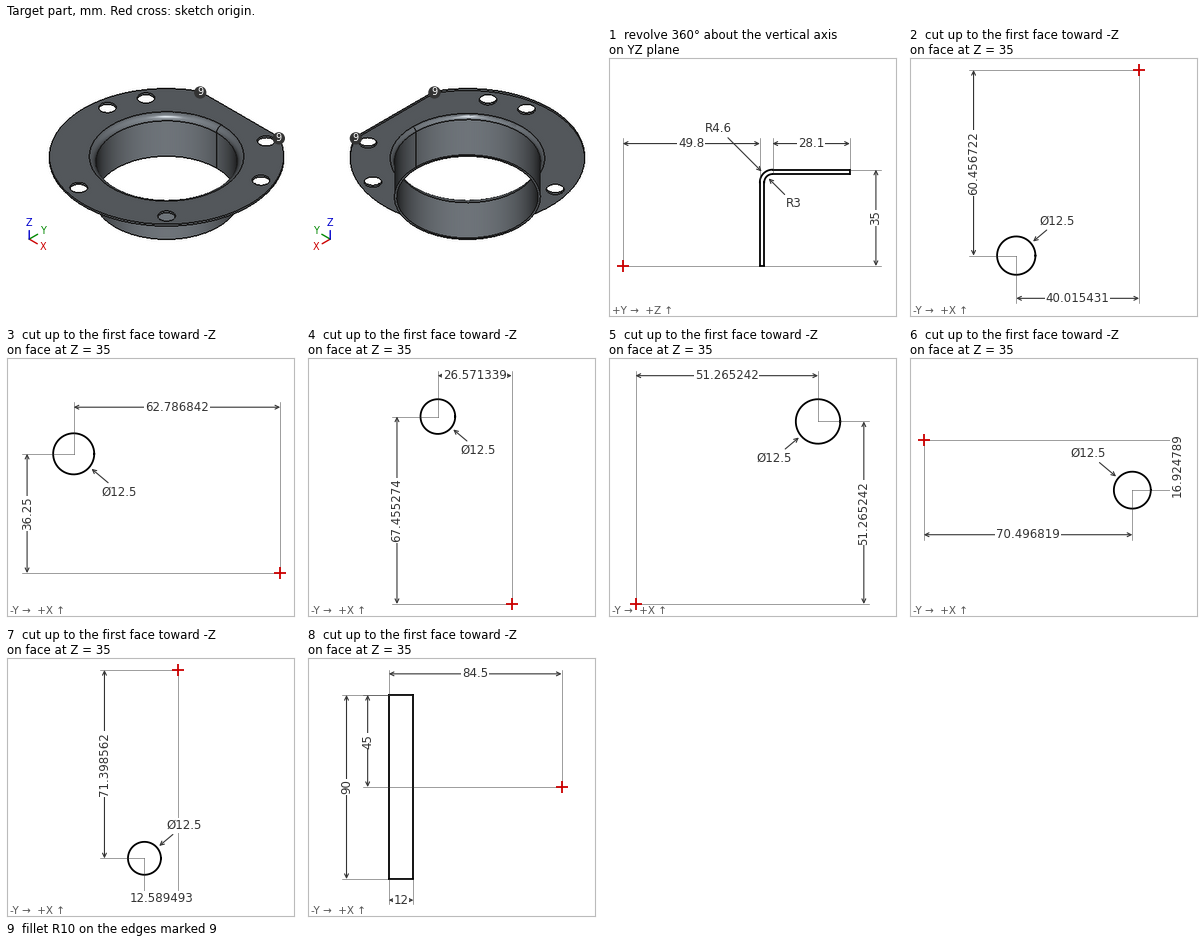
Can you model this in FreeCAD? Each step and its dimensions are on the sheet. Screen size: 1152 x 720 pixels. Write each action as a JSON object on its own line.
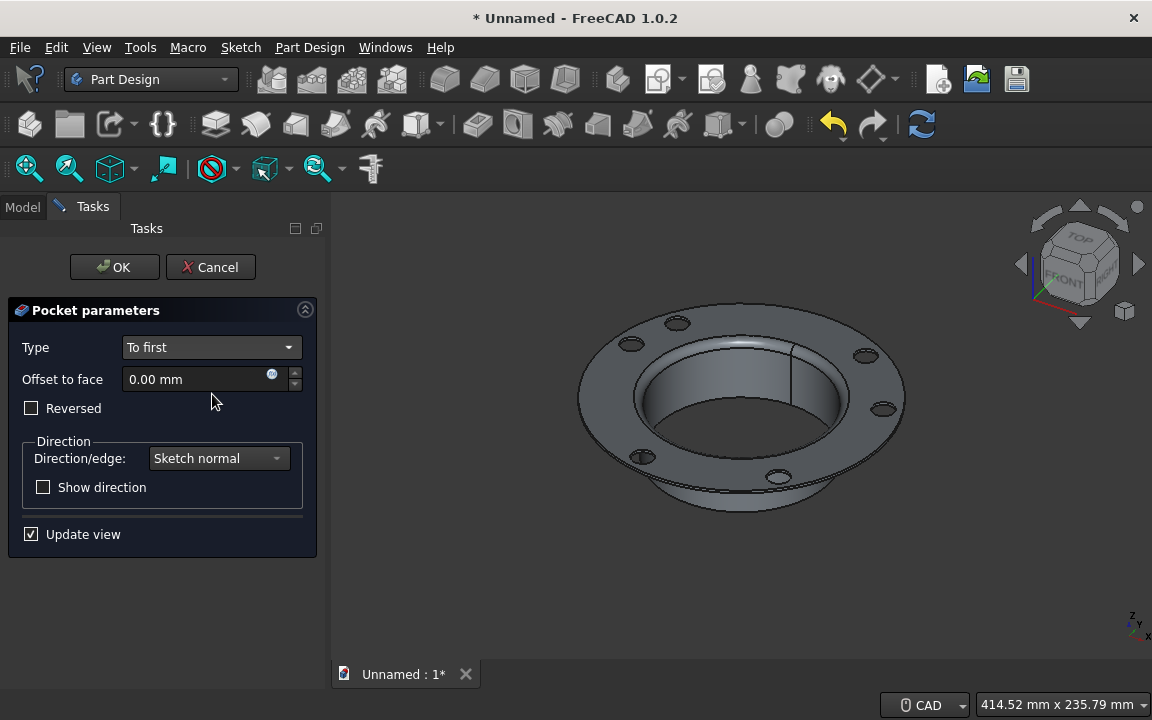
{"action": "left_click", "coordinate": [115, 267]}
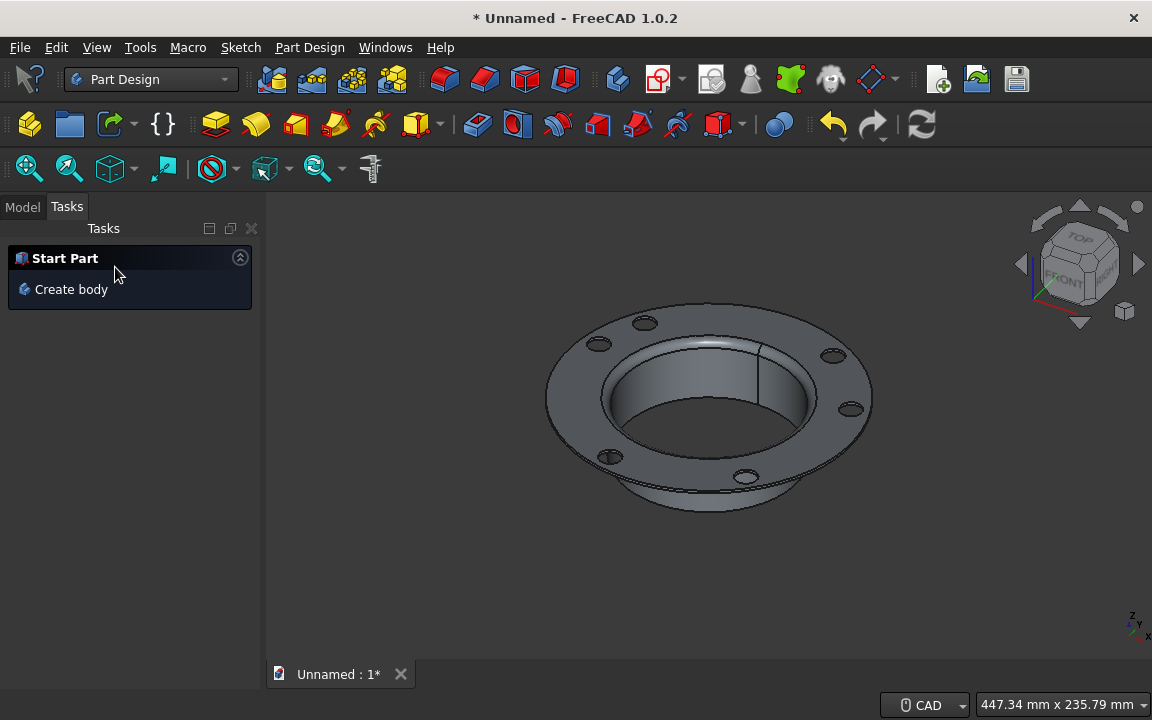
{"action": "left_click", "coordinate": [837, 377]}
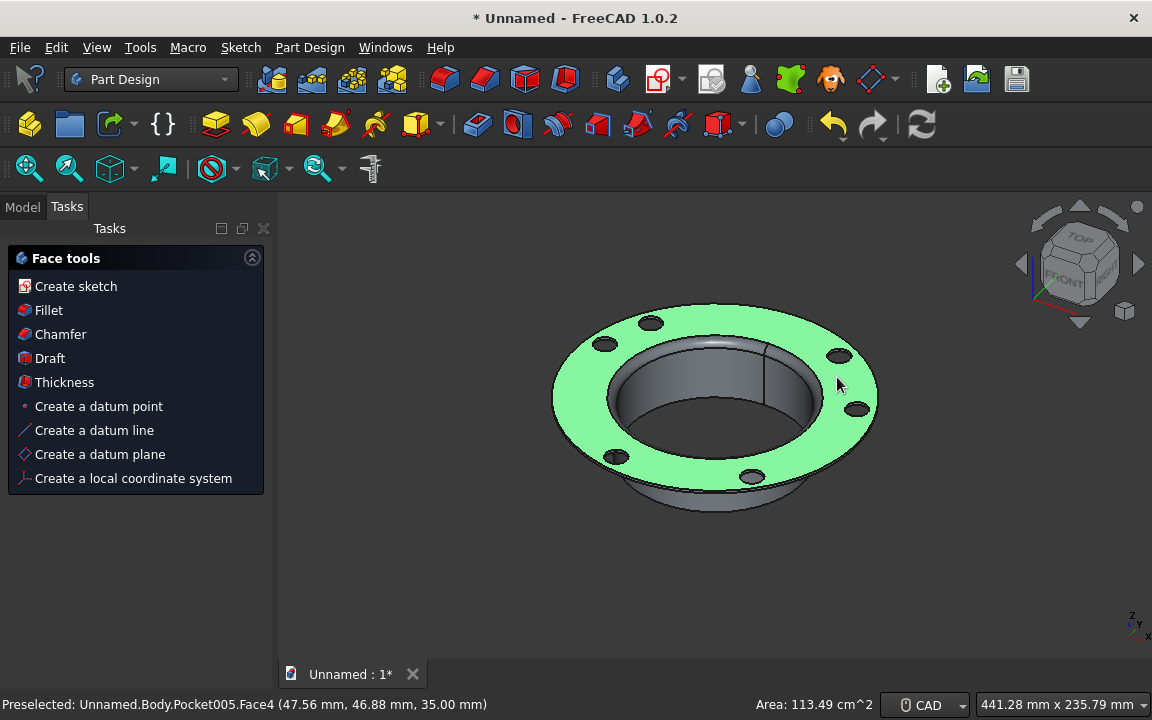
{"action": "left_click", "coordinate": [658, 80]}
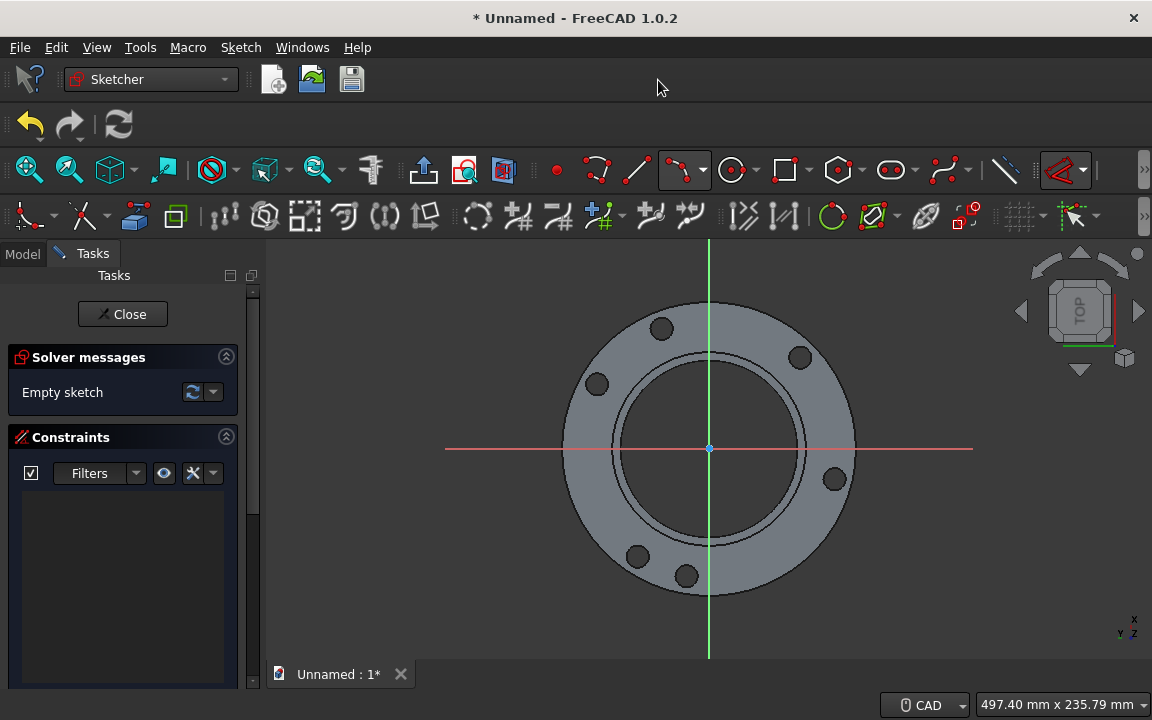
{"action": "scroll", "coordinate": [620, 449], "scroll_direction": "up", "scroll_amount": 2}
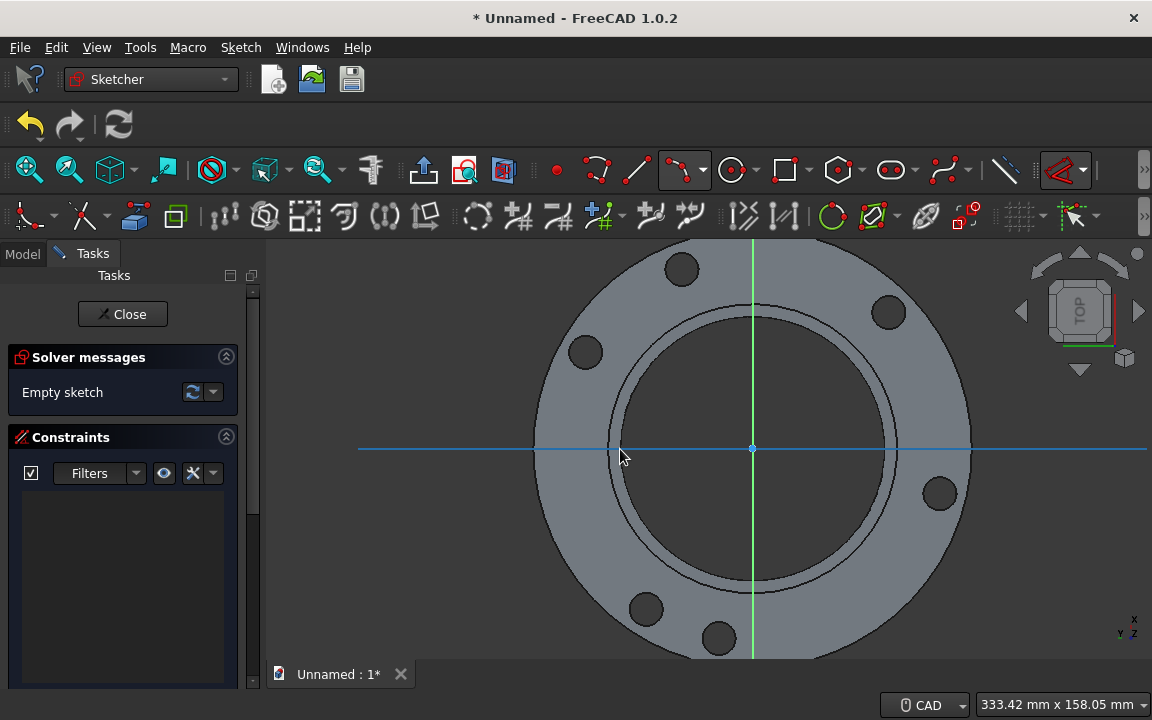
{"action": "key", "text": "g r"}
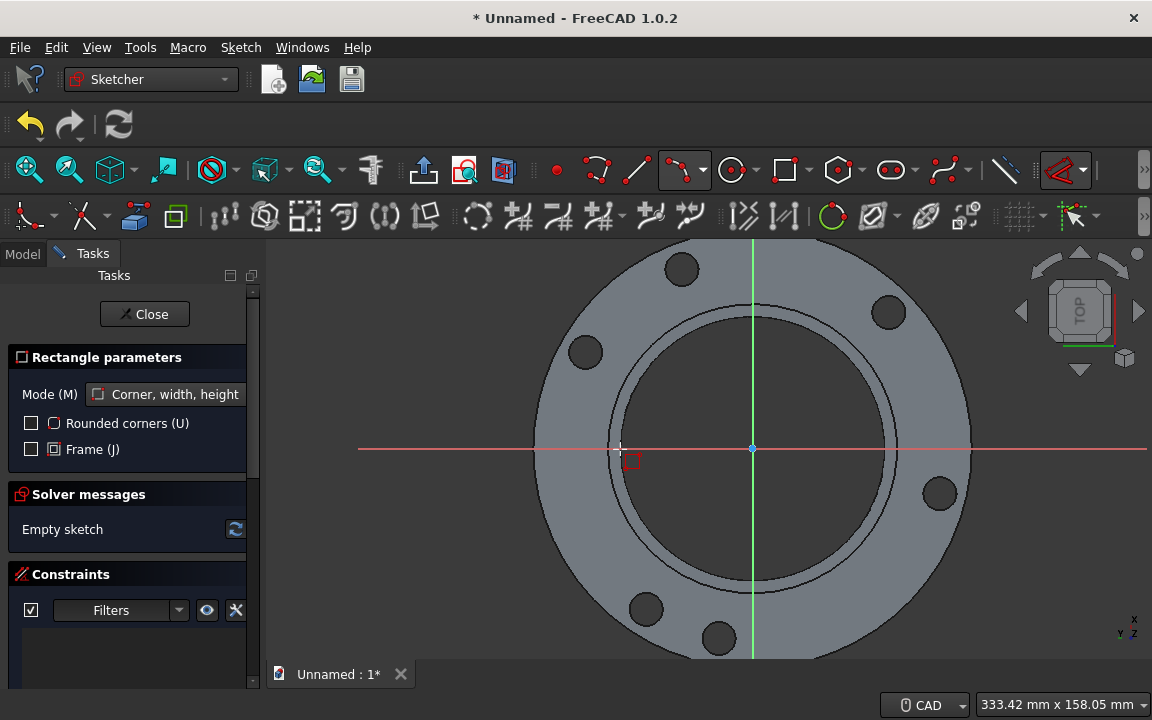
{"action": "left_click", "coordinate": [528, 329]}
{"action": "mouse_move", "coordinate": [560, 568]}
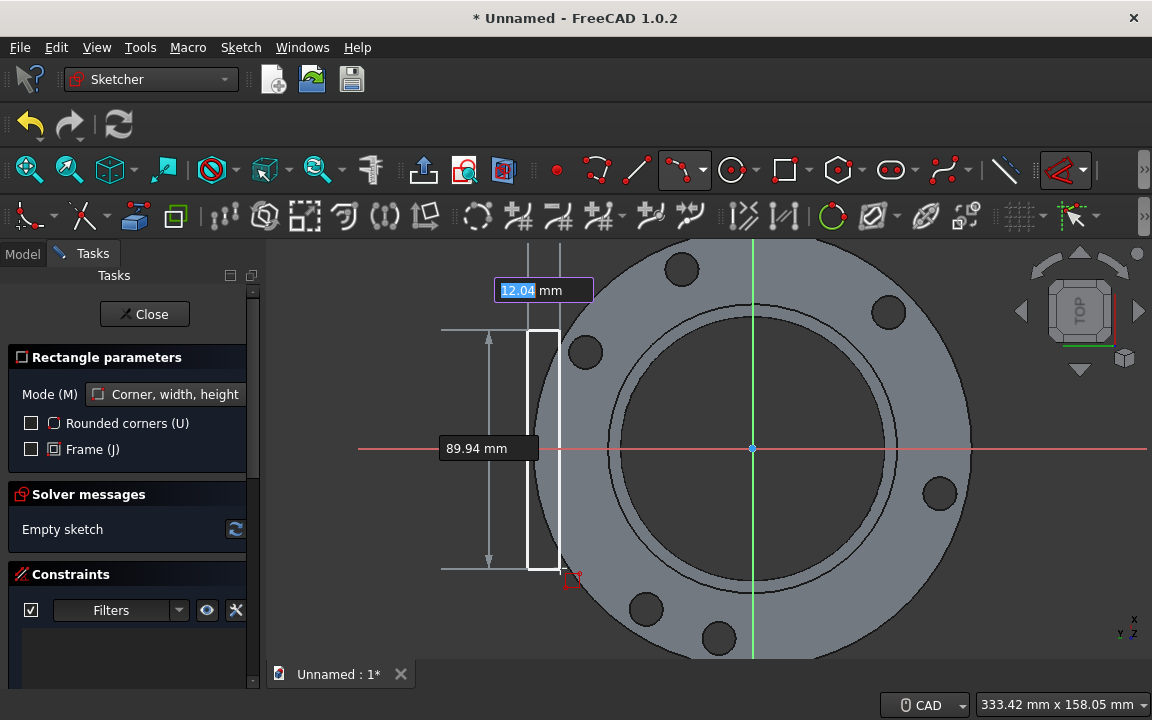
{"action": "type", "text": "12"}
{"action": "key", "text": "Tab"}
{"action": "type", "text": "90"}
{"action": "key", "text": "Return"}
{"action": "key", "text": "Escape"}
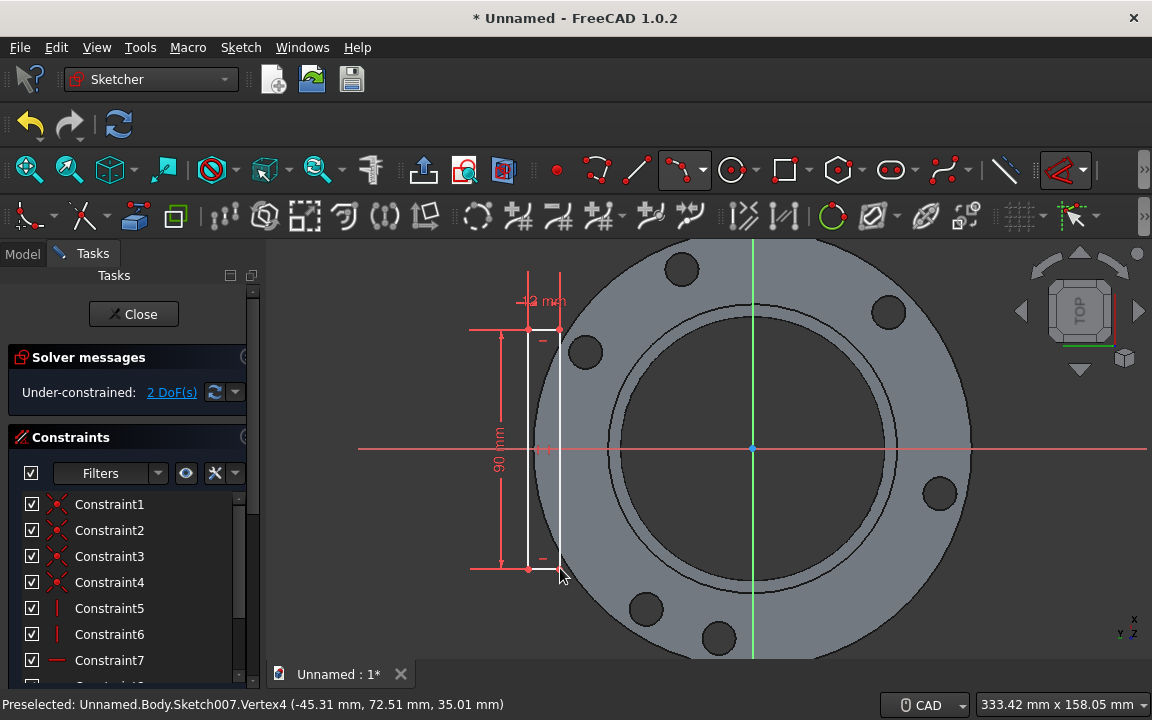
{"action": "left_click", "coordinate": [528, 330]}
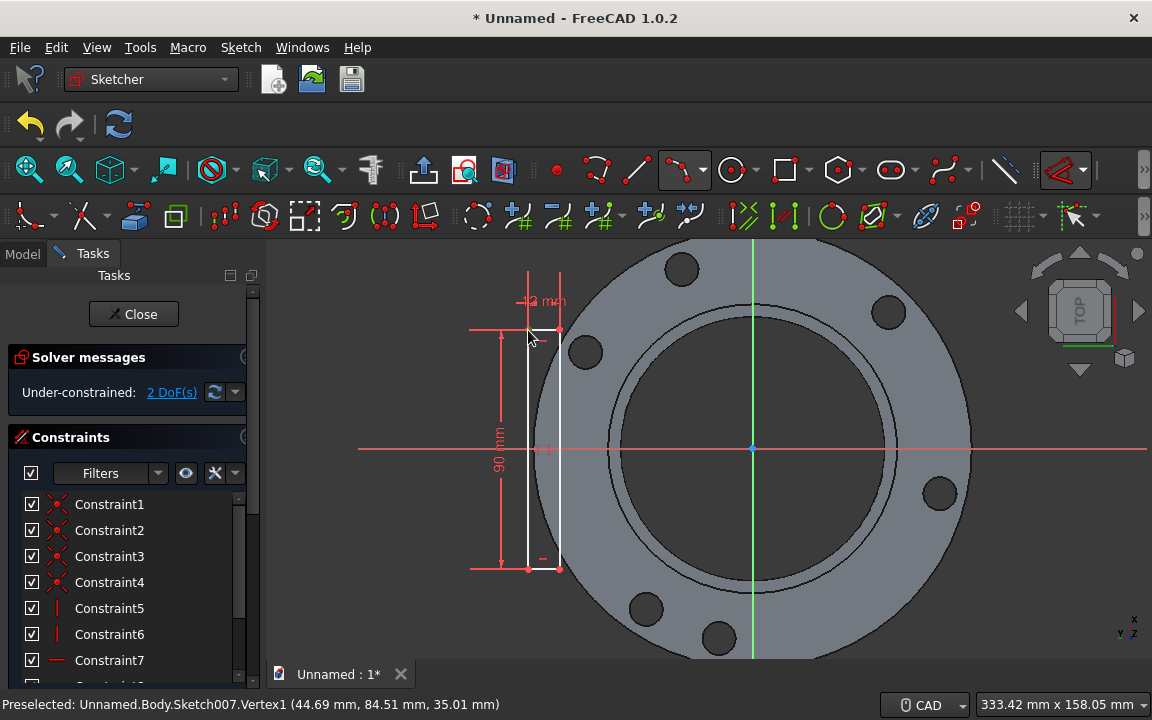
{"action": "left_click", "coordinate": [1086, 170]}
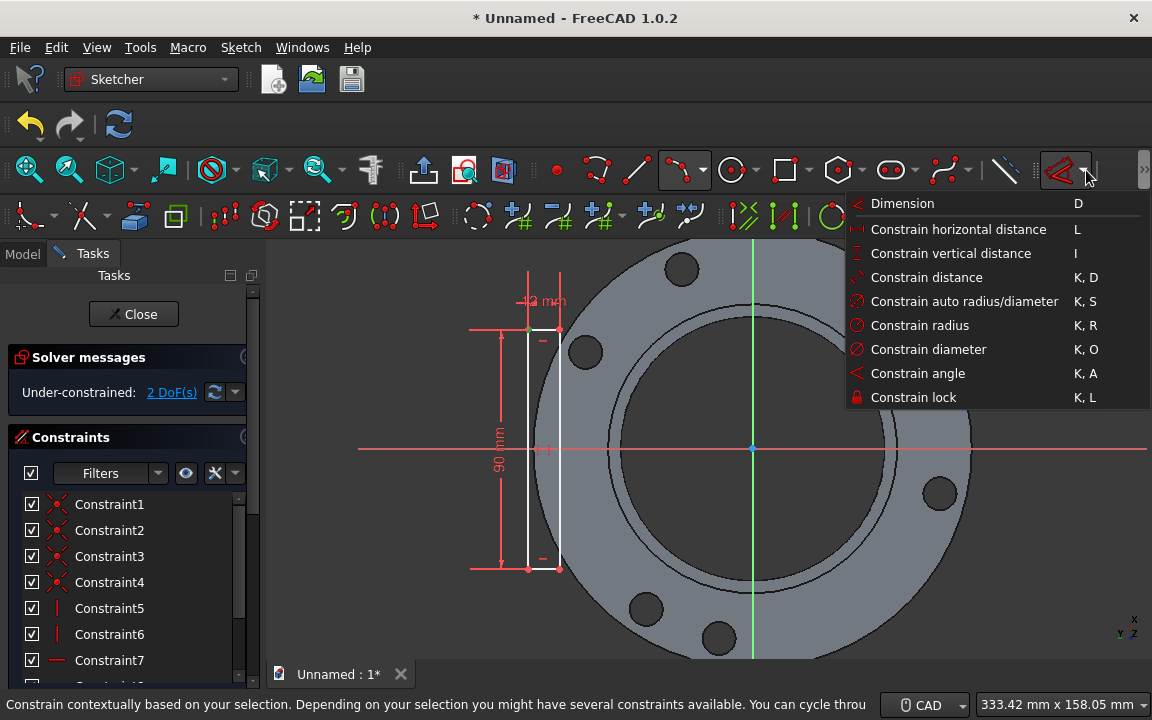
{"action": "left_click", "coordinate": [998, 253]}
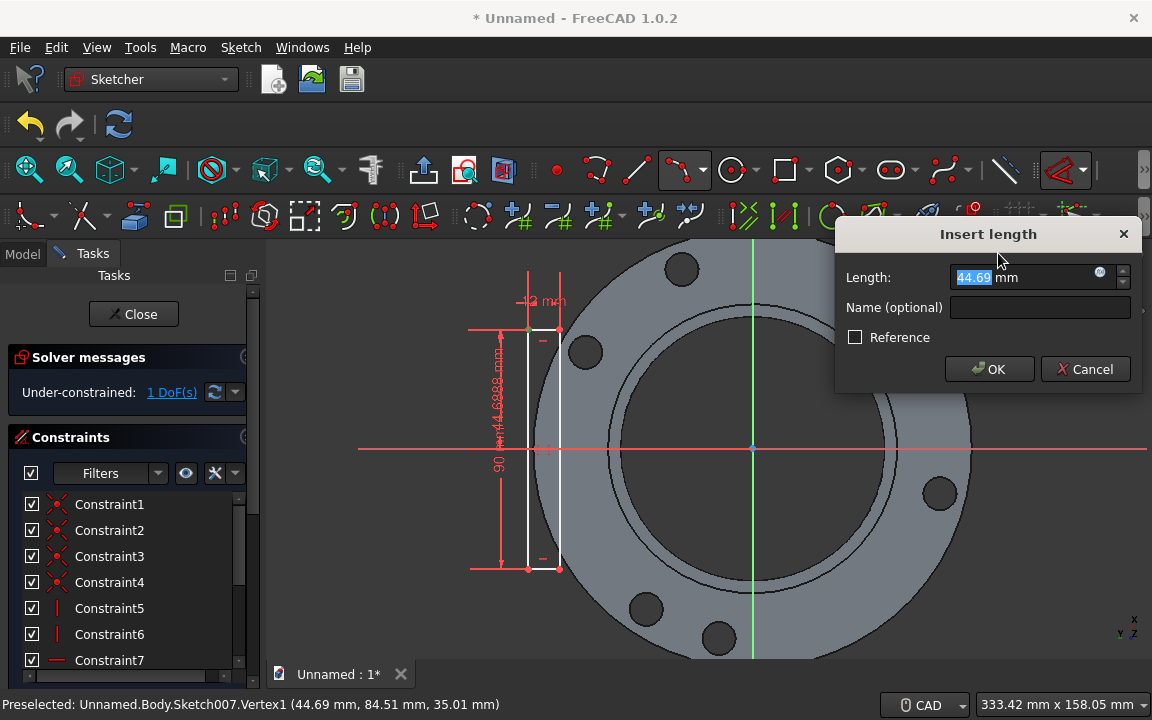
{"action": "type", "text": "45"}
{"action": "key", "text": "Return"}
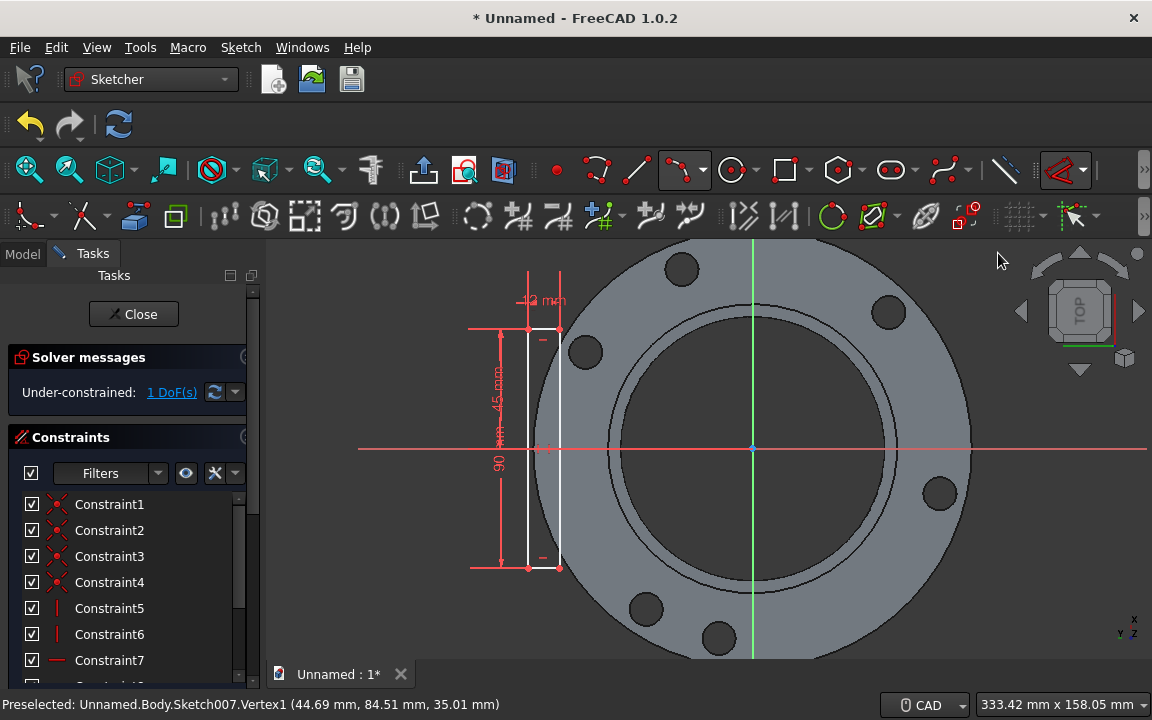
{"action": "left_click", "coordinate": [528, 329]}